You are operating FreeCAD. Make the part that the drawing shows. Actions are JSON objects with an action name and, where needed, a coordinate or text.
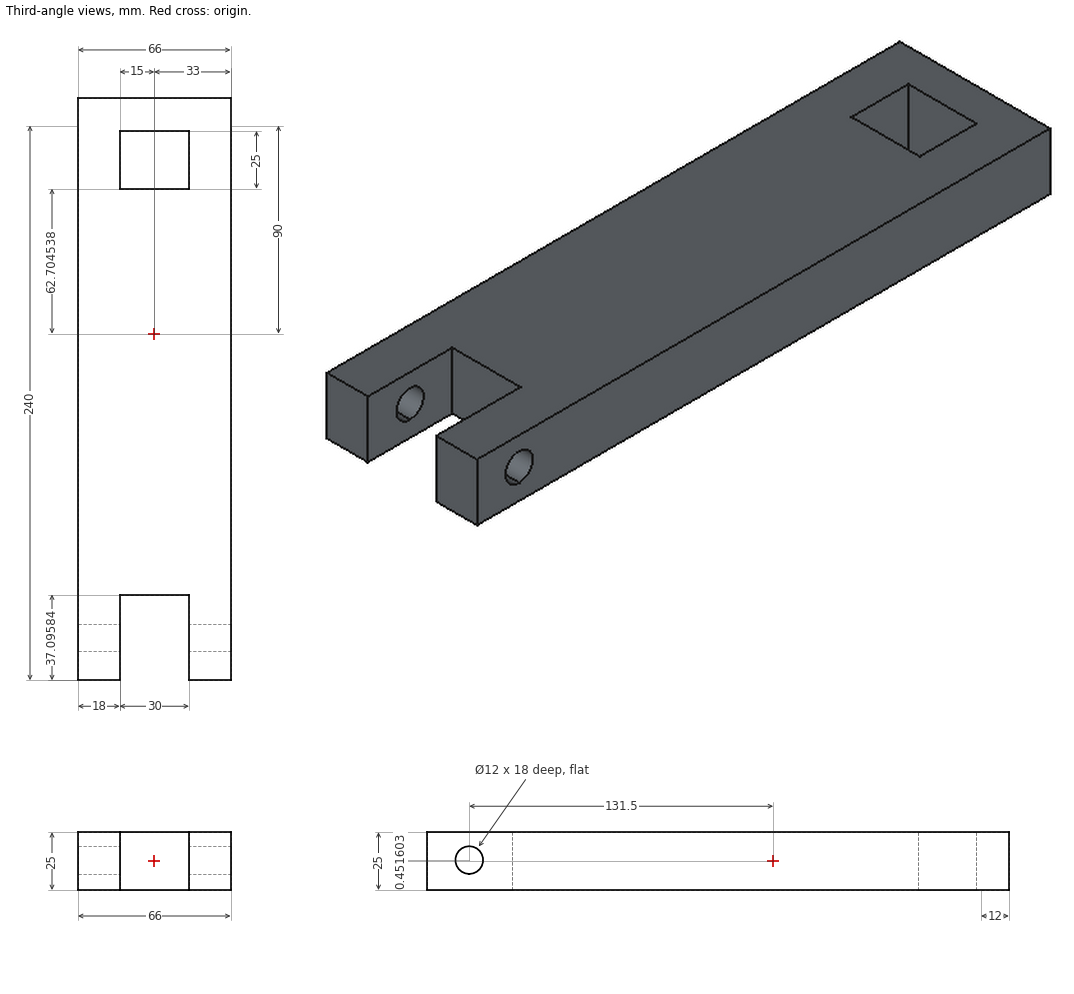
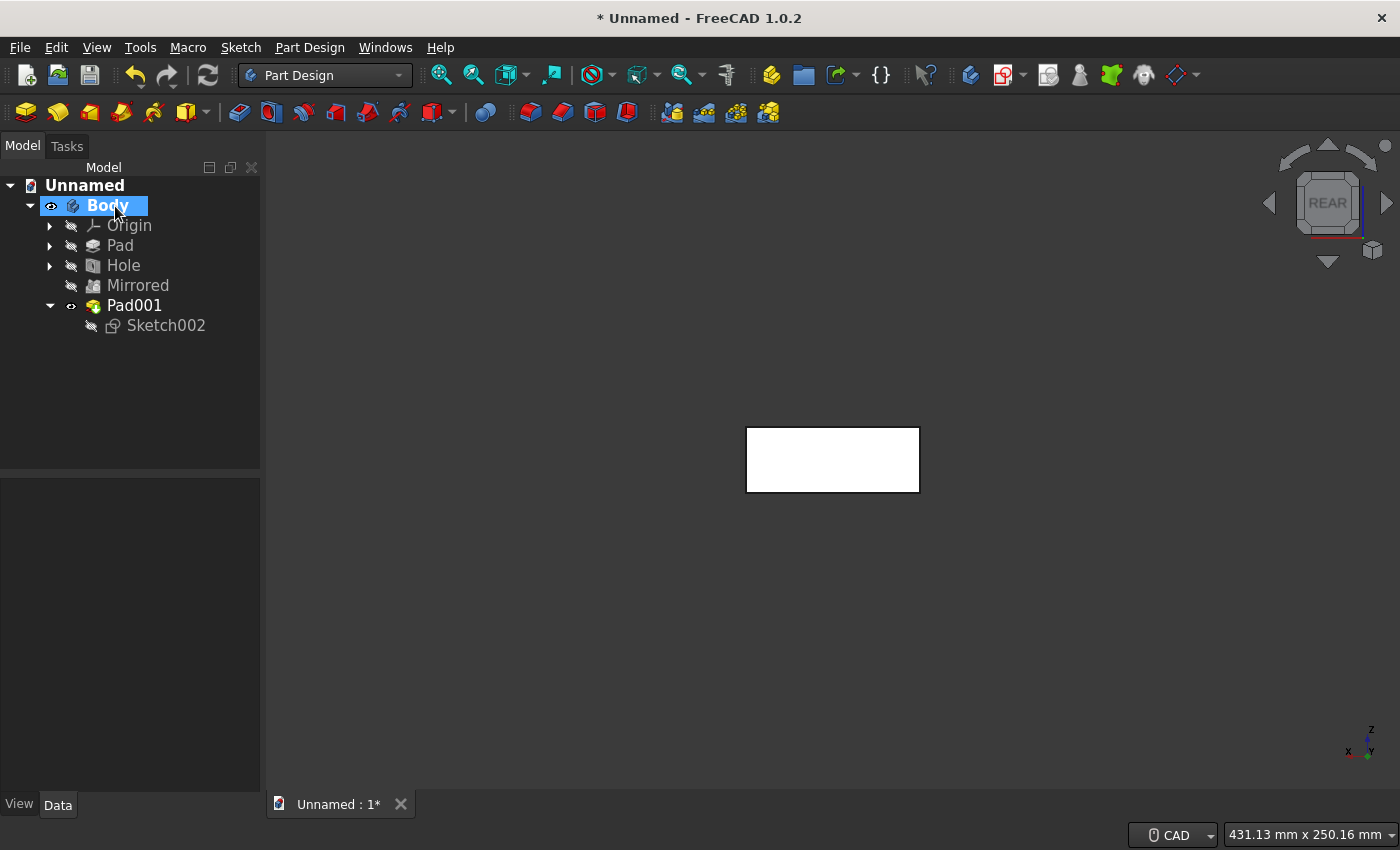
{"action": "left_click", "coordinate": [442, 76]}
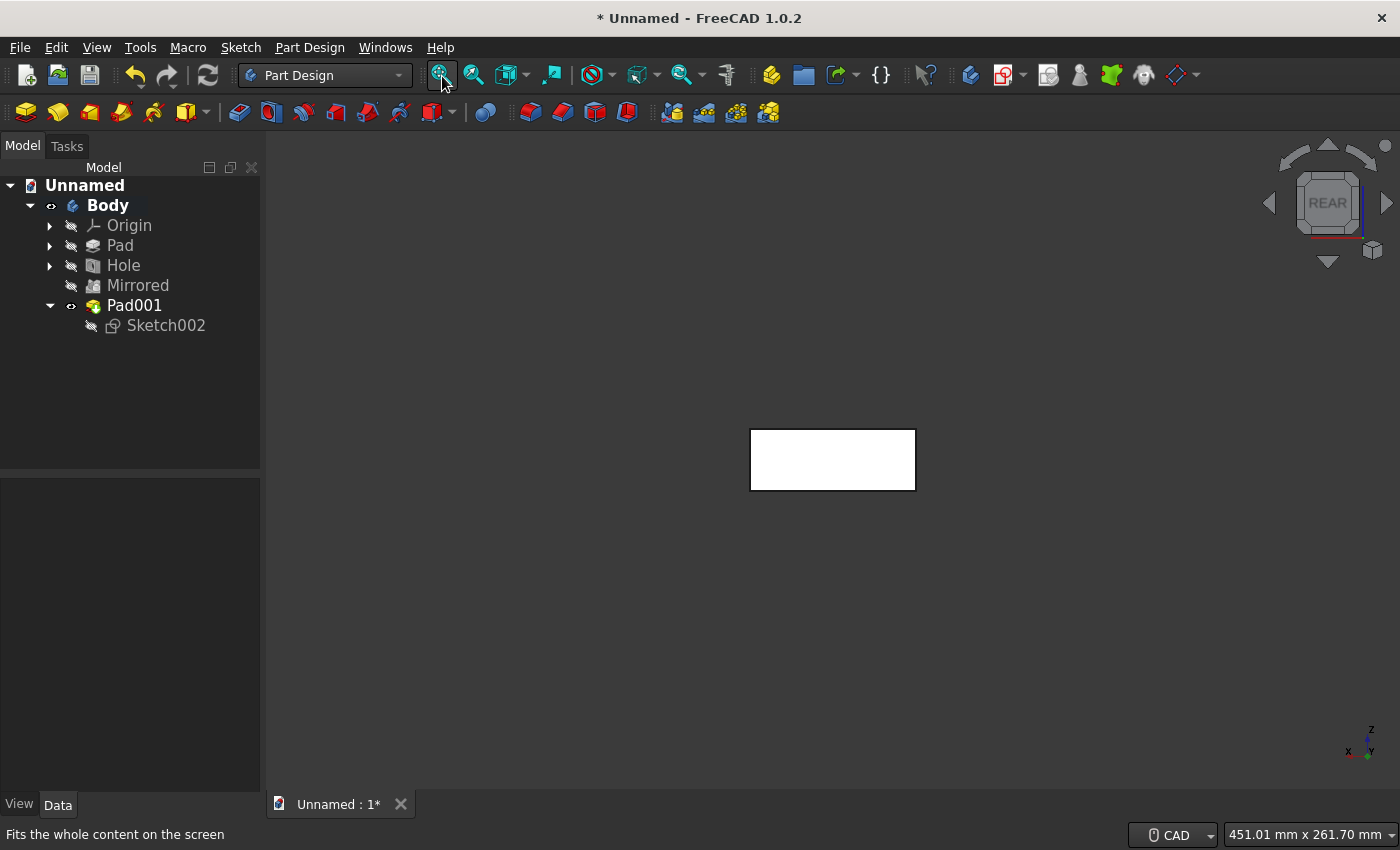
{"action": "key", "text": "5"}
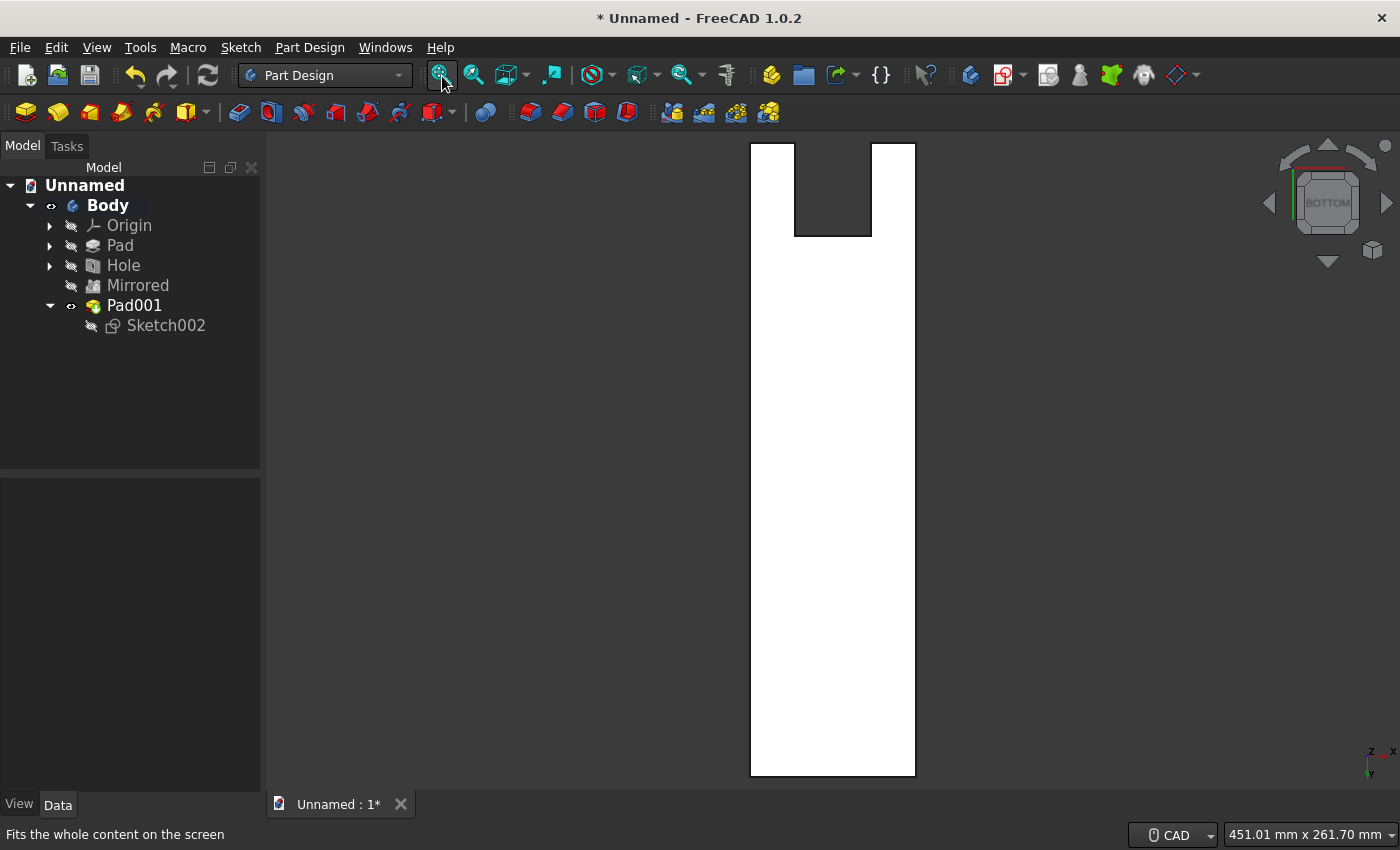
{"action": "left_click", "coordinate": [833, 640]}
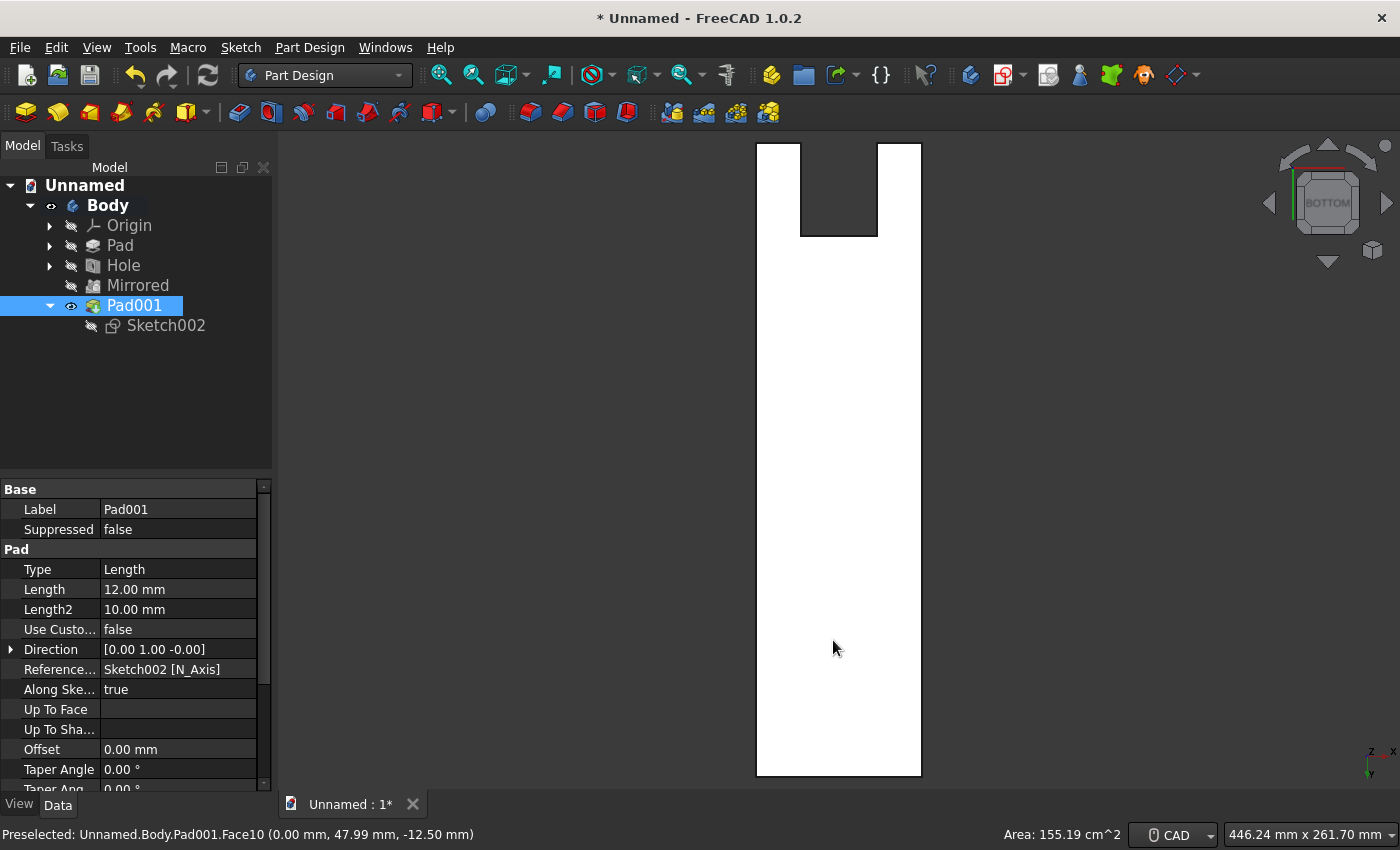
{"action": "left_click", "coordinate": [1004, 76]}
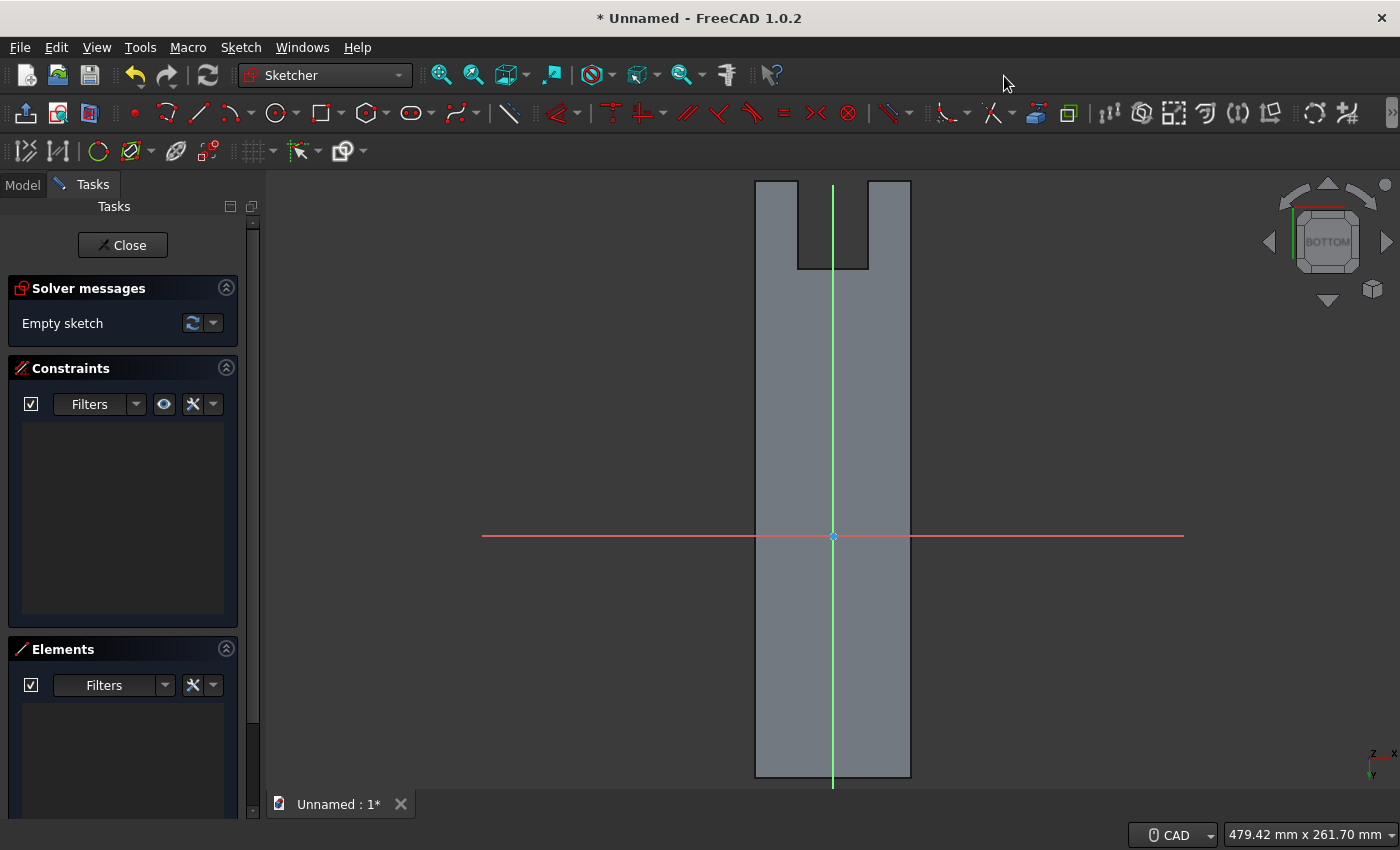
{"action": "scroll", "coordinate": [844, 751], "scroll_direction": "up", "scroll_amount": 10}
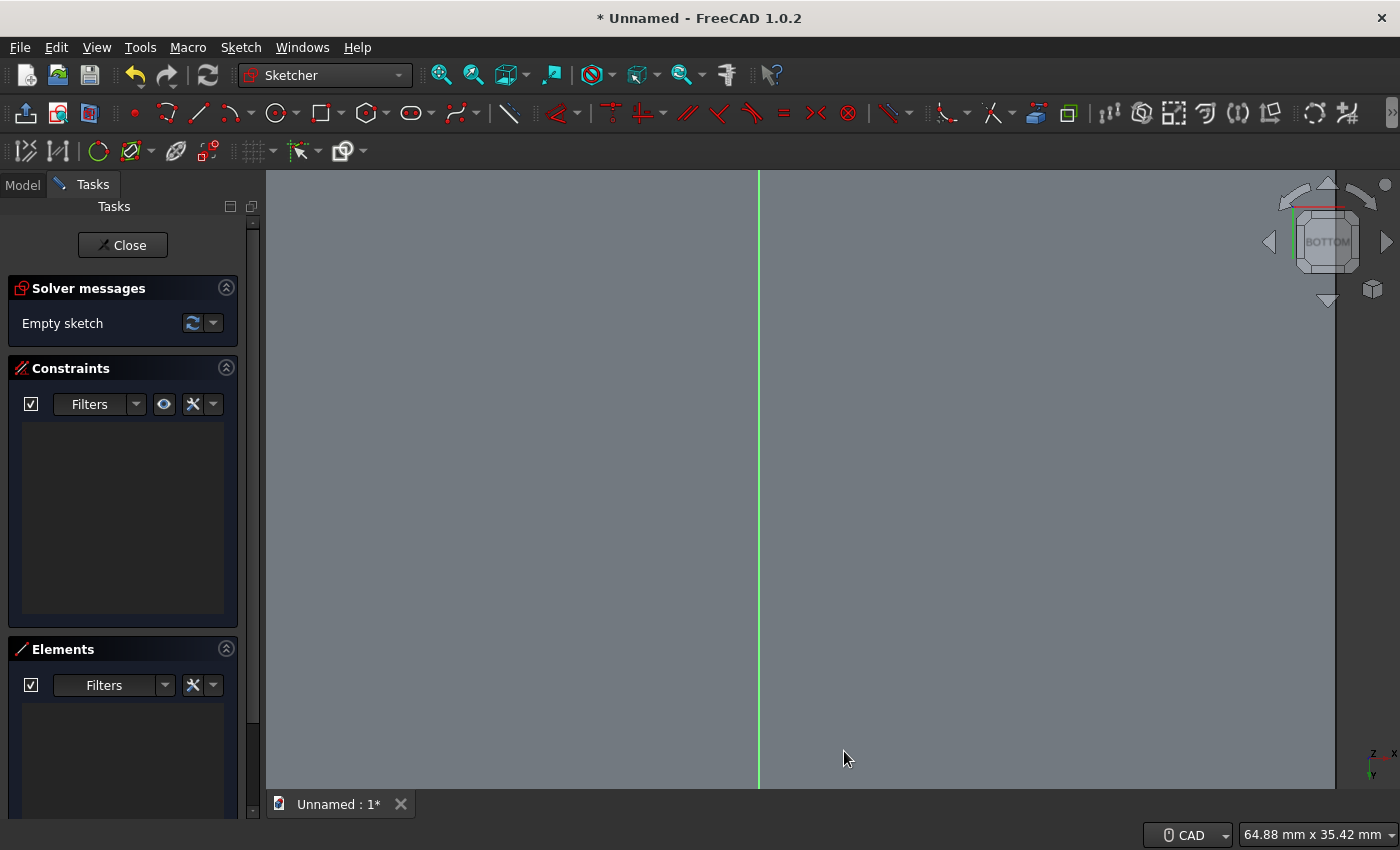
{"action": "left_click", "coordinate": [322, 114]}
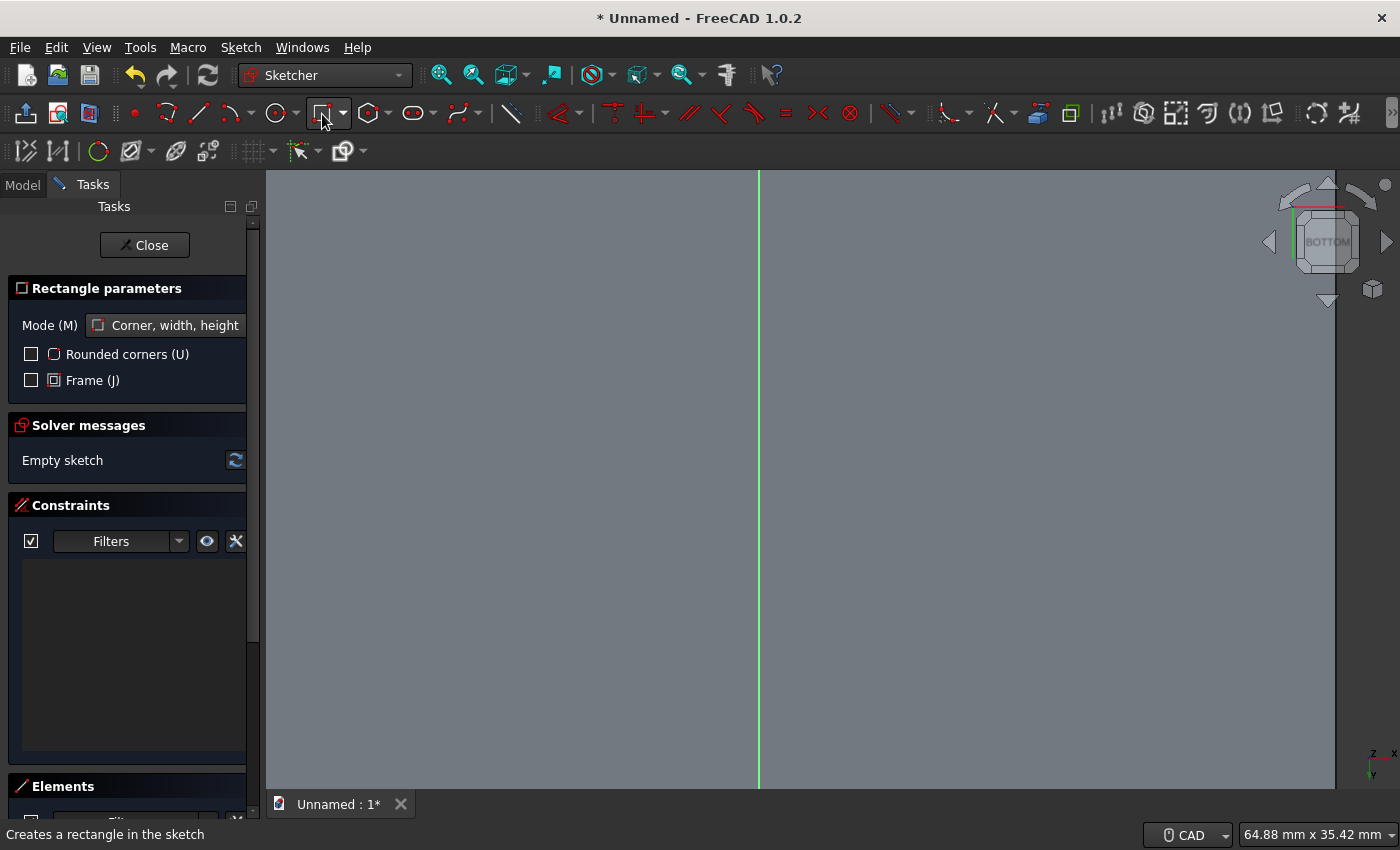
{"action": "left_click", "coordinate": [497, 254]}
{"action": "mouse_move", "coordinate": [1022, 691]}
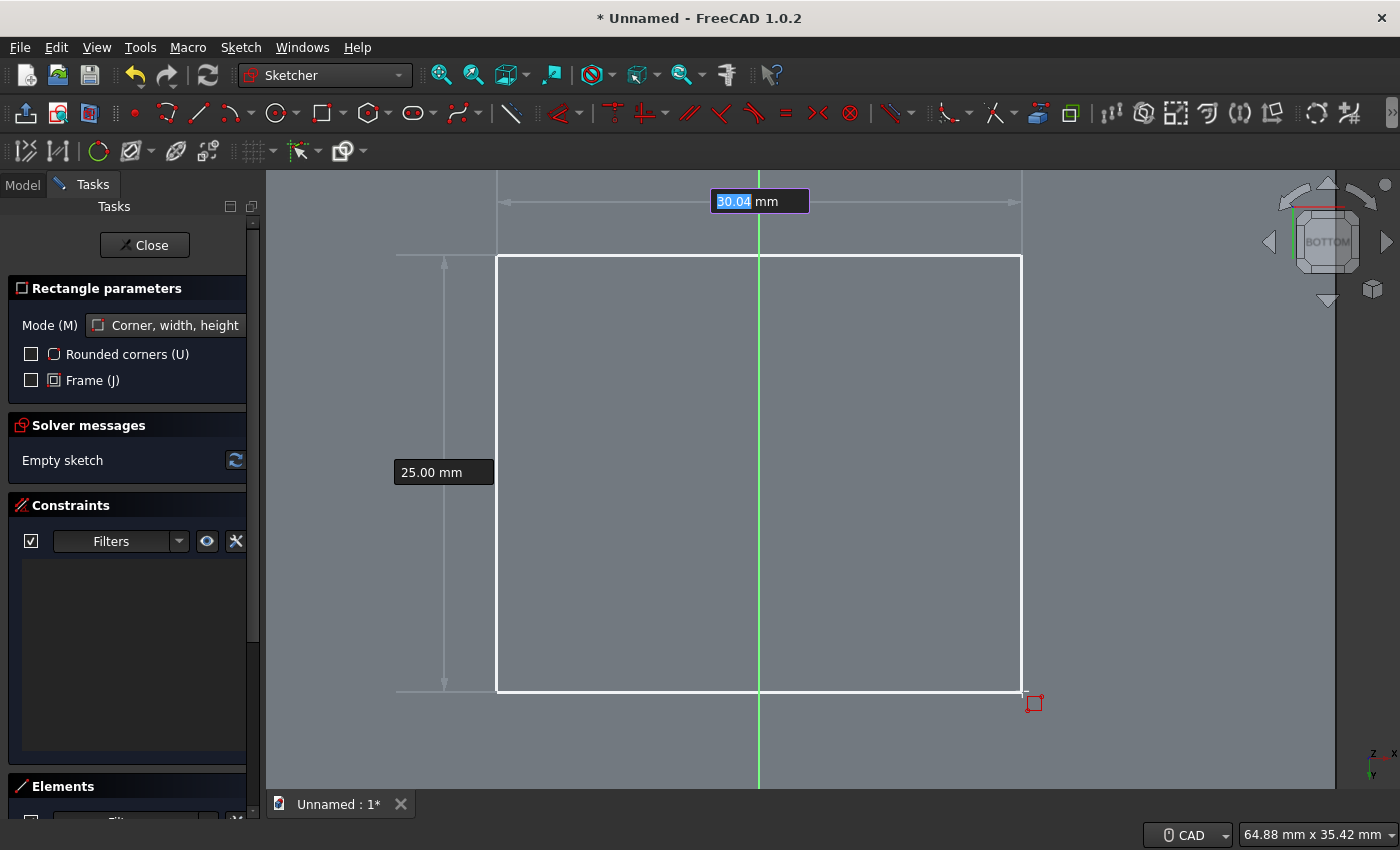
{"action": "type", "text": "30"}
{"action": "key", "text": "Tab"}
{"action": "type", "text": "25"}
{"action": "key", "text": "Return"}
{"action": "key", "text": "Escape"}